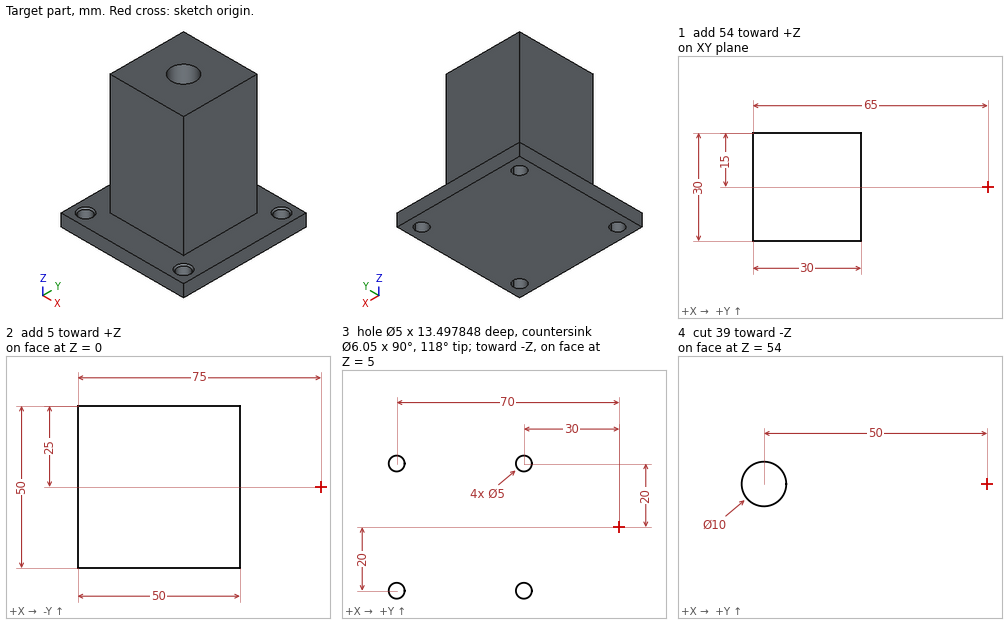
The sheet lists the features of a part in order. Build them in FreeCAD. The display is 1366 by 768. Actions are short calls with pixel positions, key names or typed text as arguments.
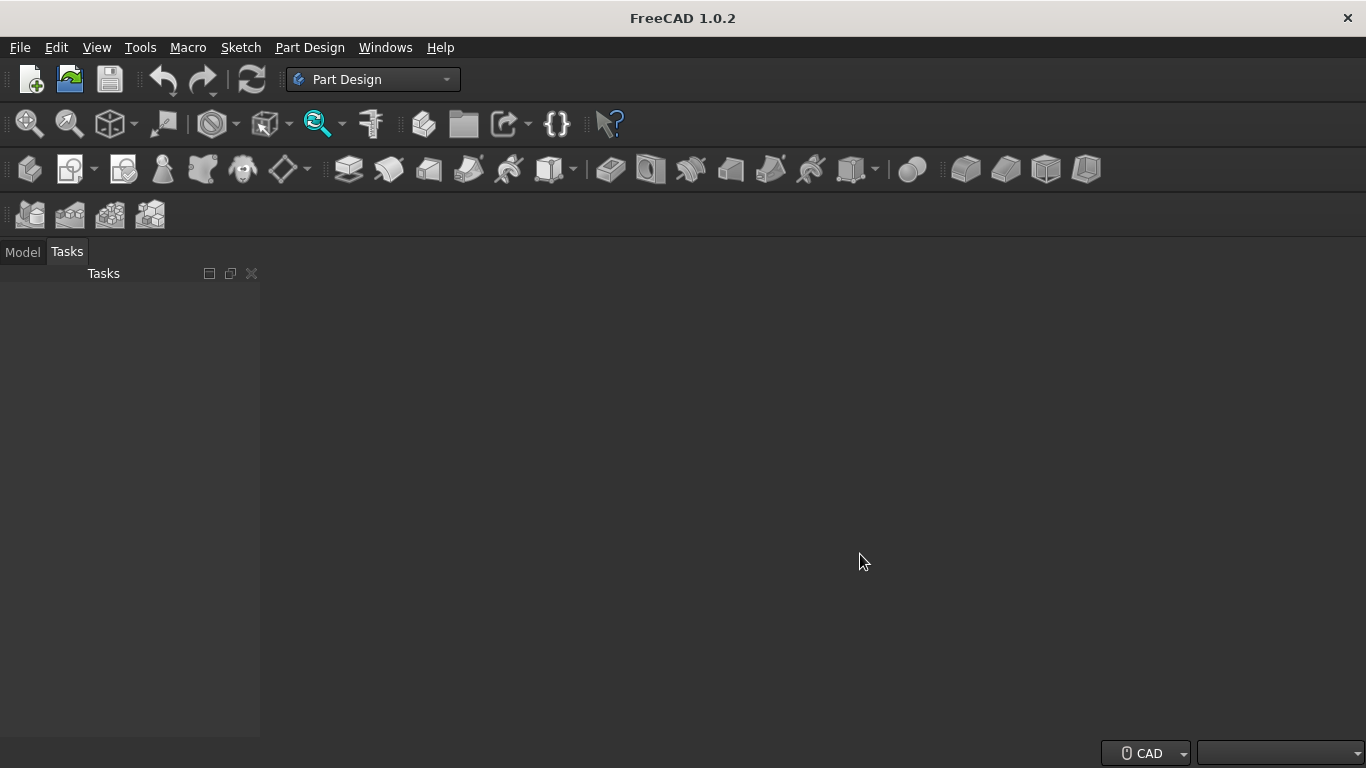
key(ctrl+n)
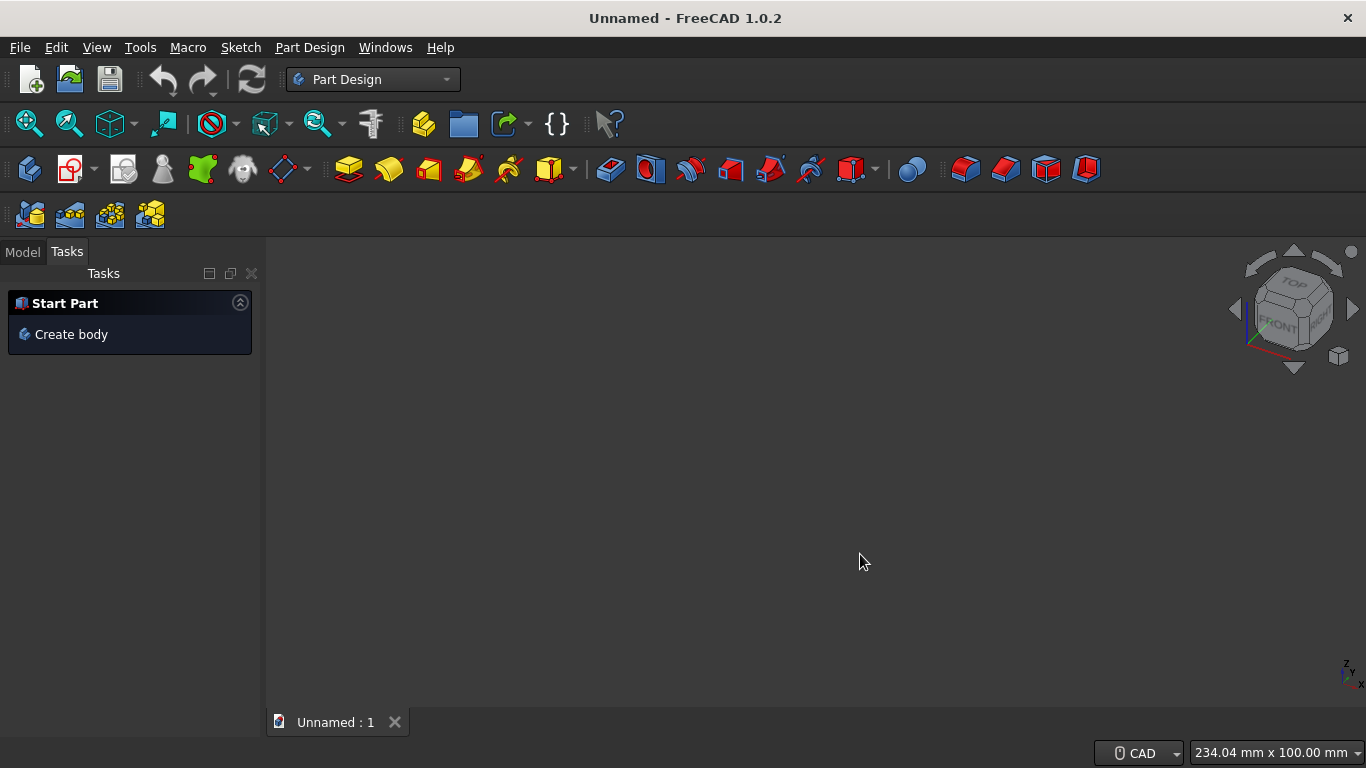
click(70, 170)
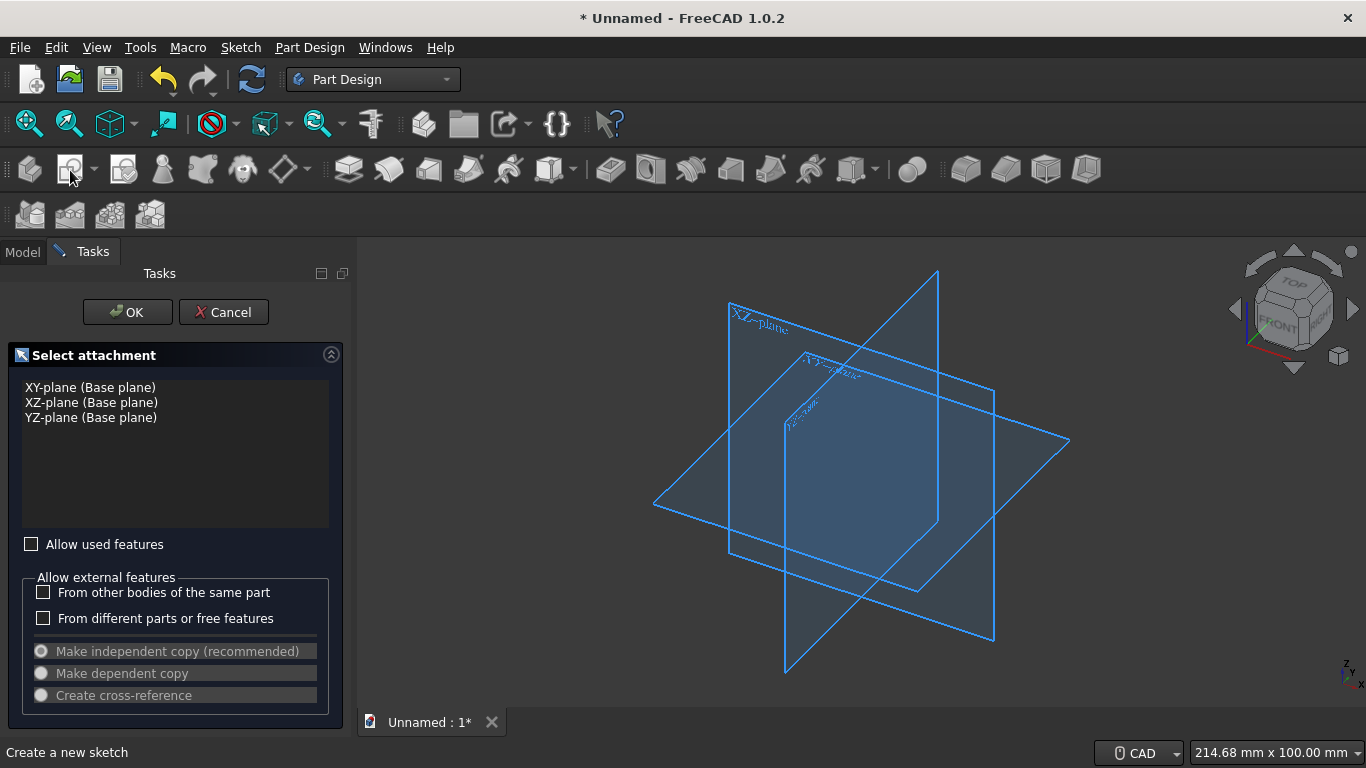
click(82, 388)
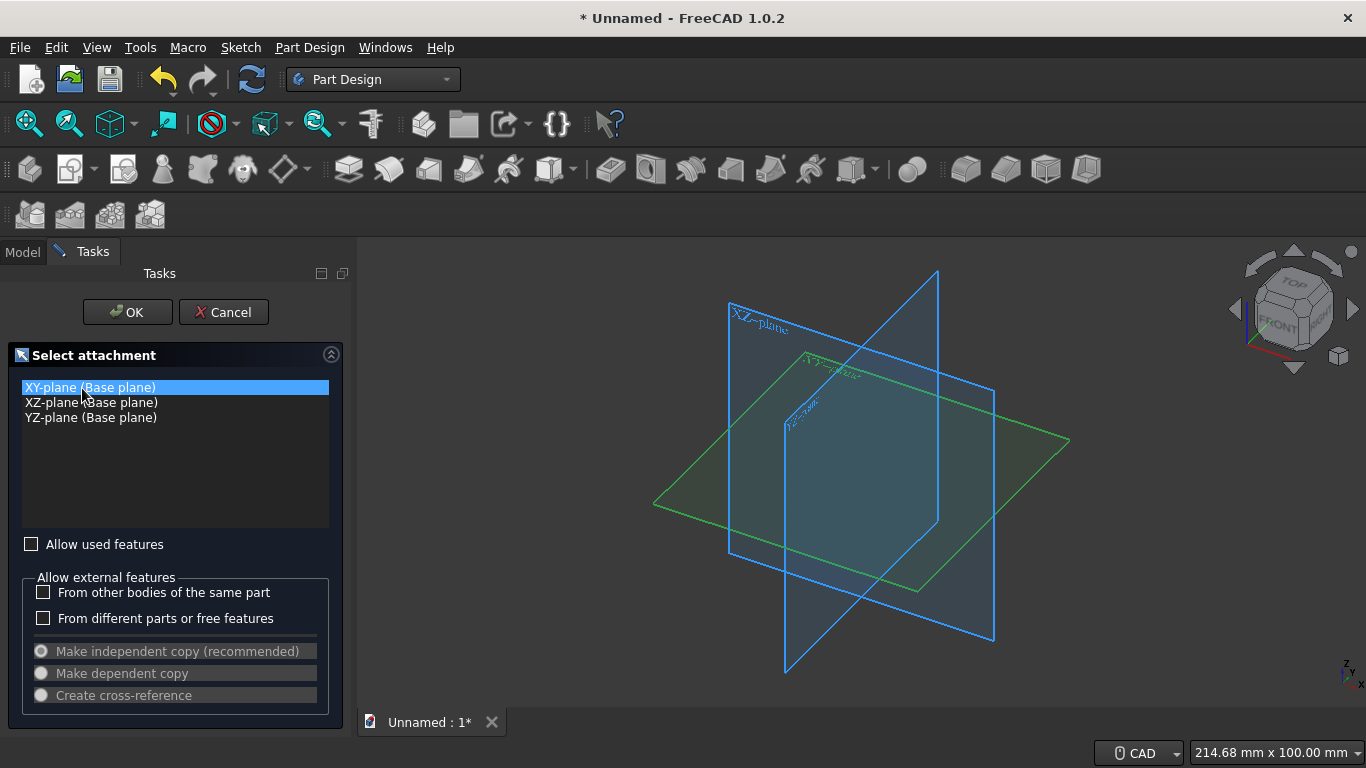
click(128, 312)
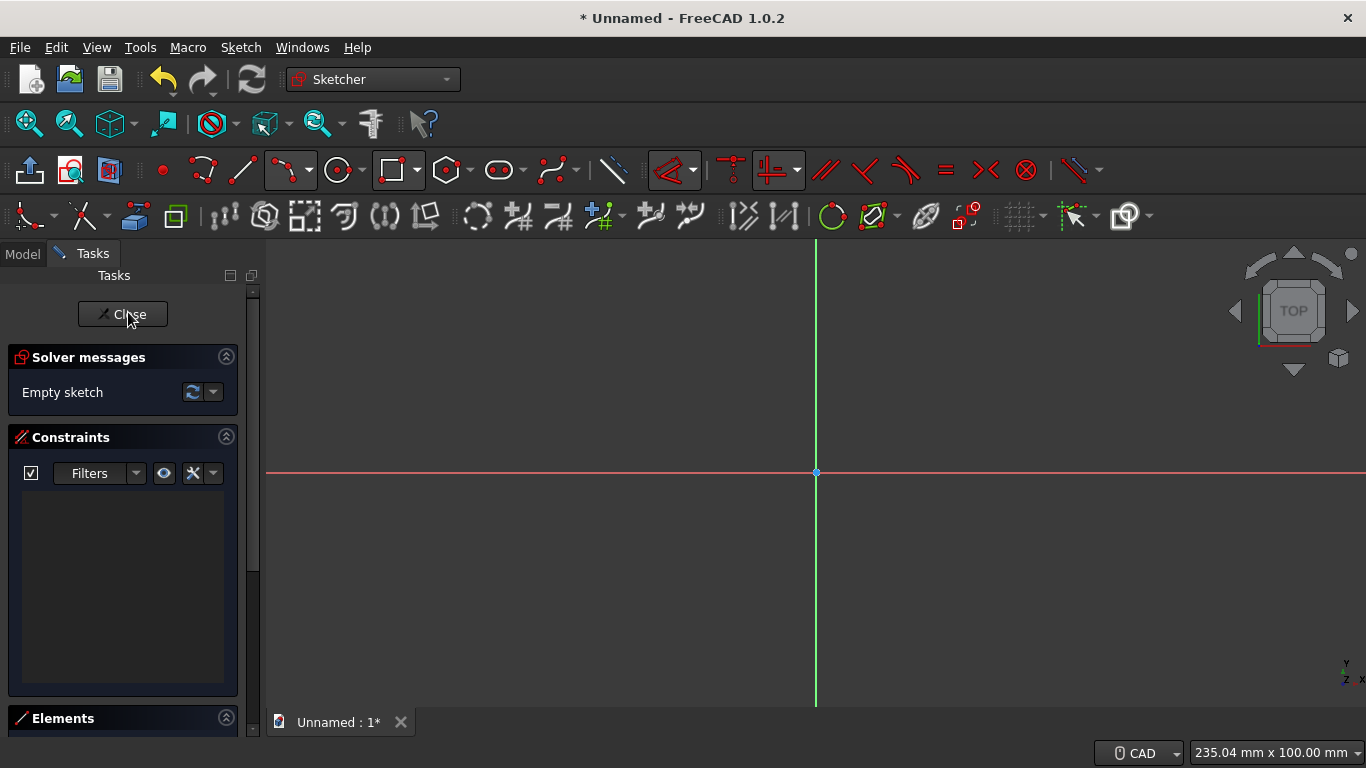
scroll(596, 473, up, 4)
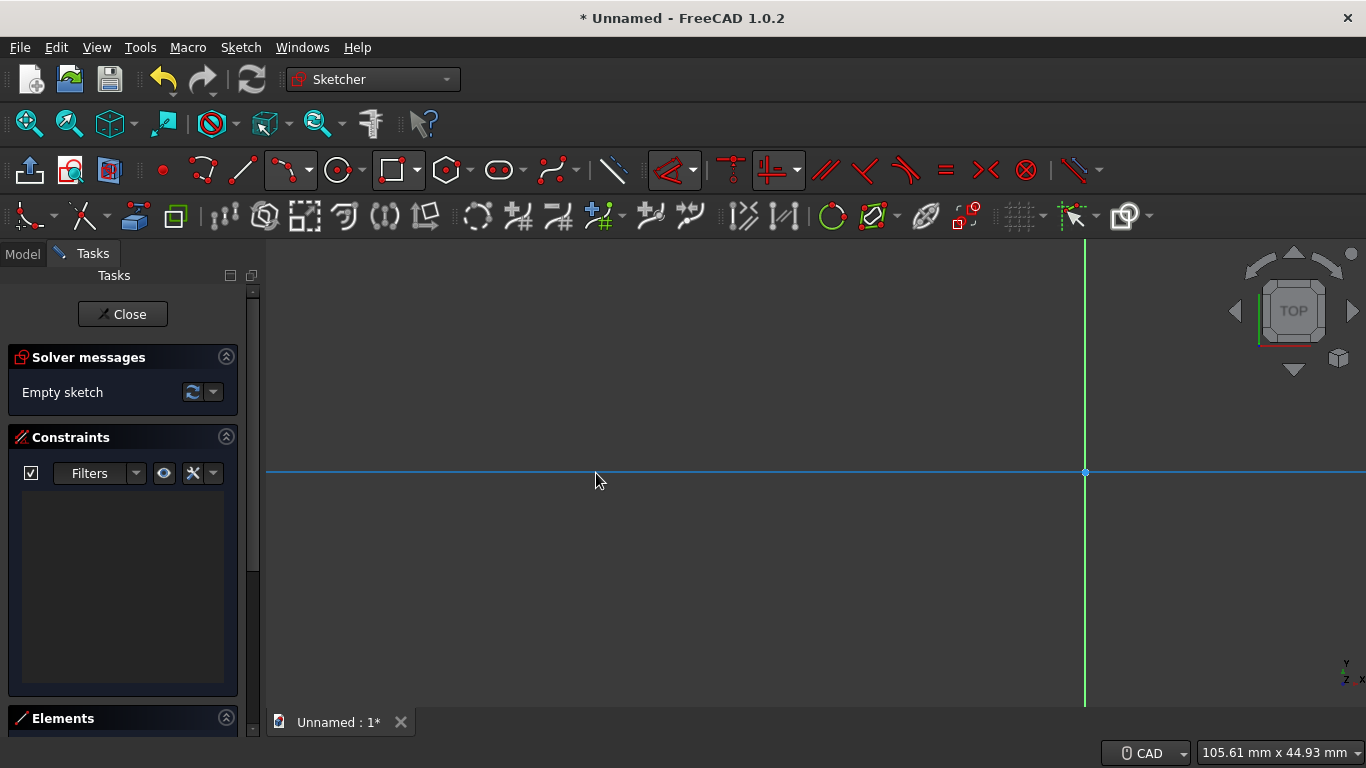
key(g)
key(r)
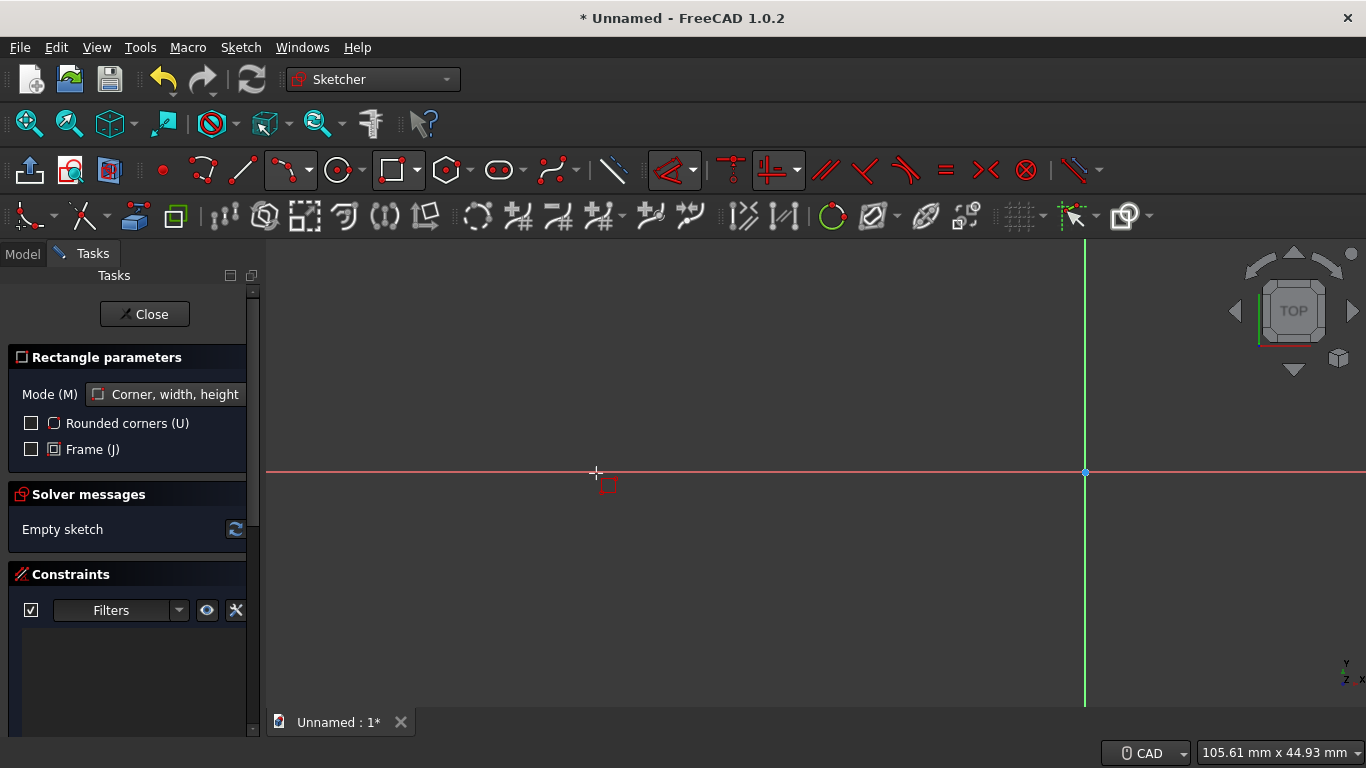
click(408, 316)
click(721, 629)
key(Escape)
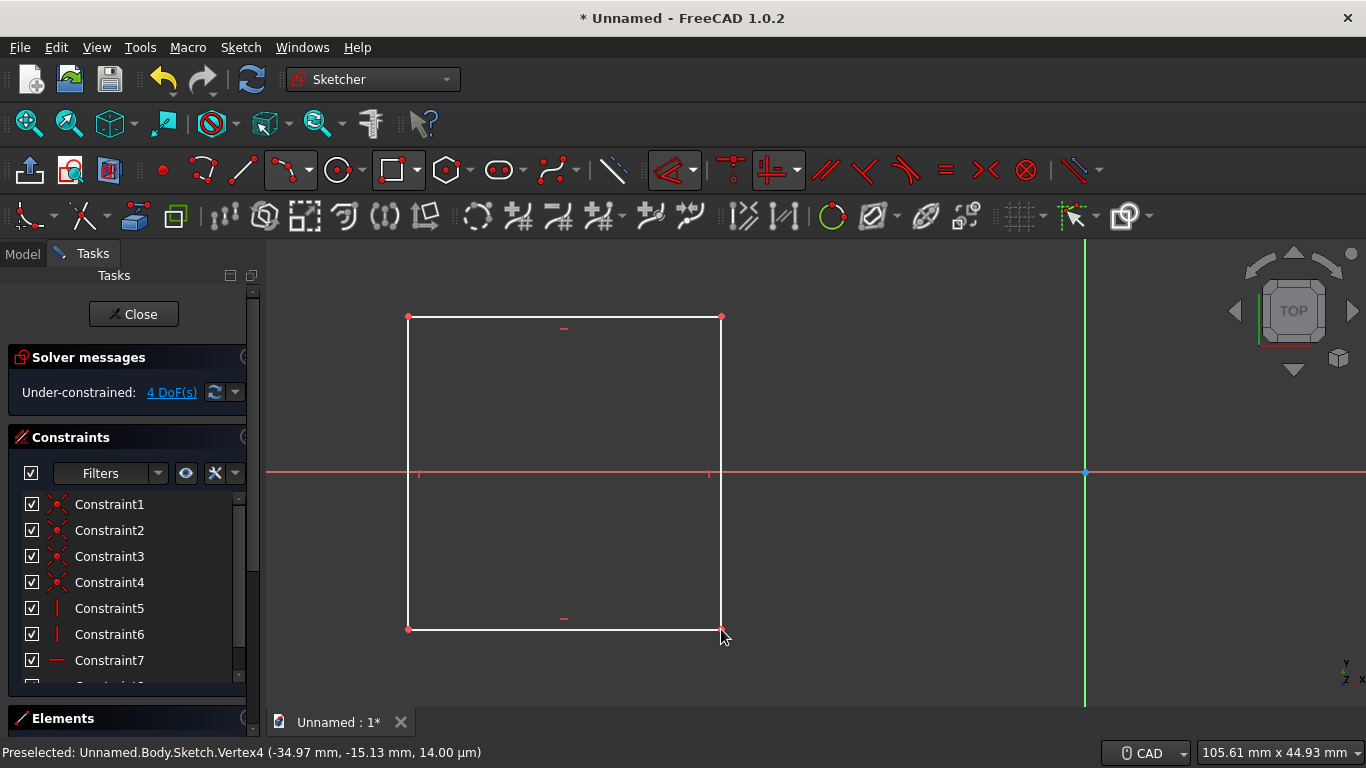
key(d)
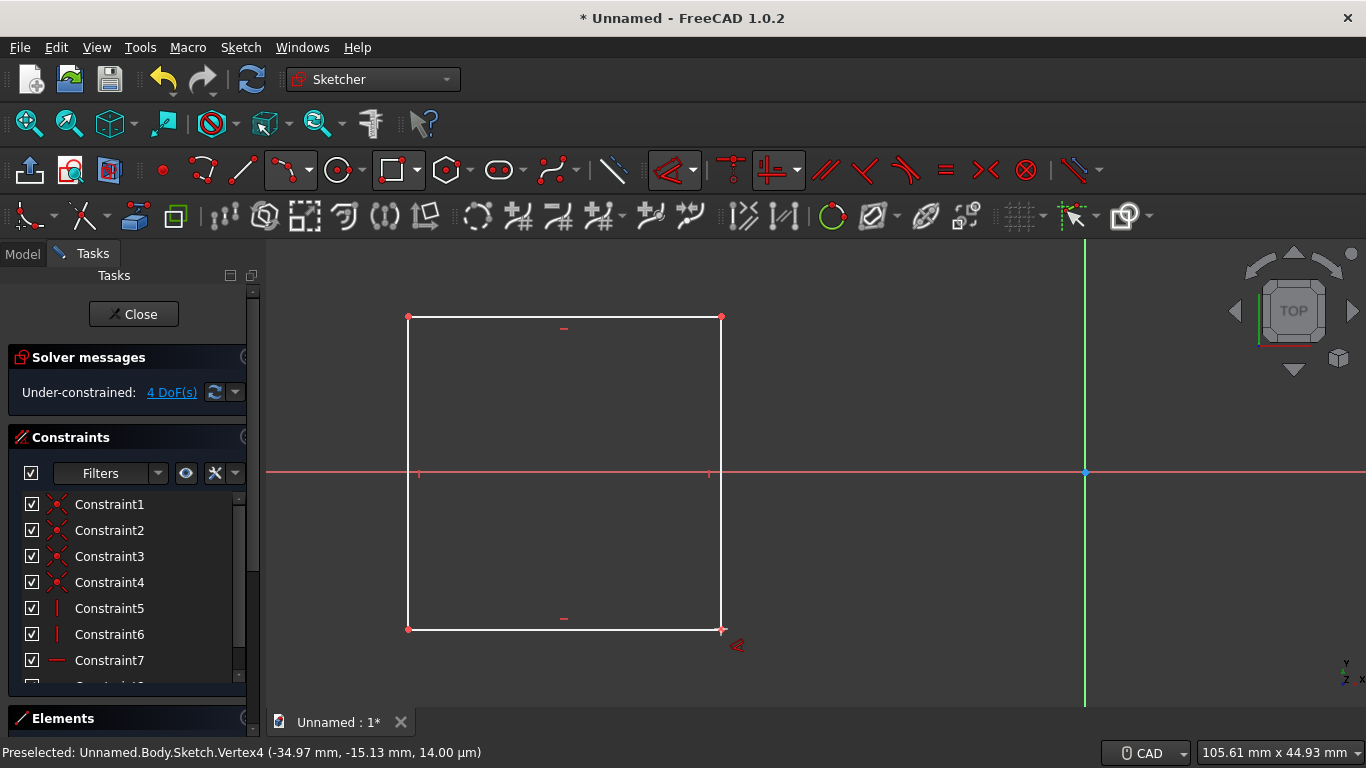
click(408, 411)
click(374, 402)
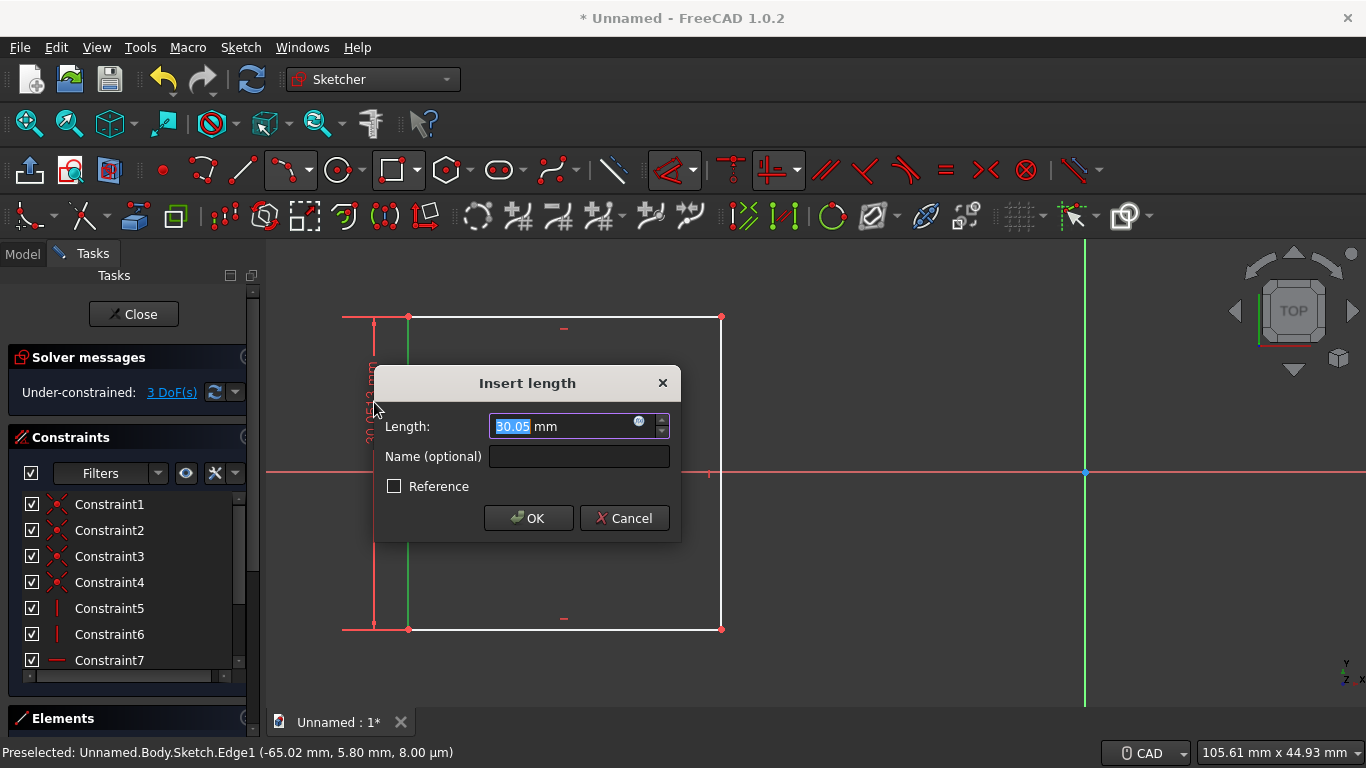
text(30)
key(Return)